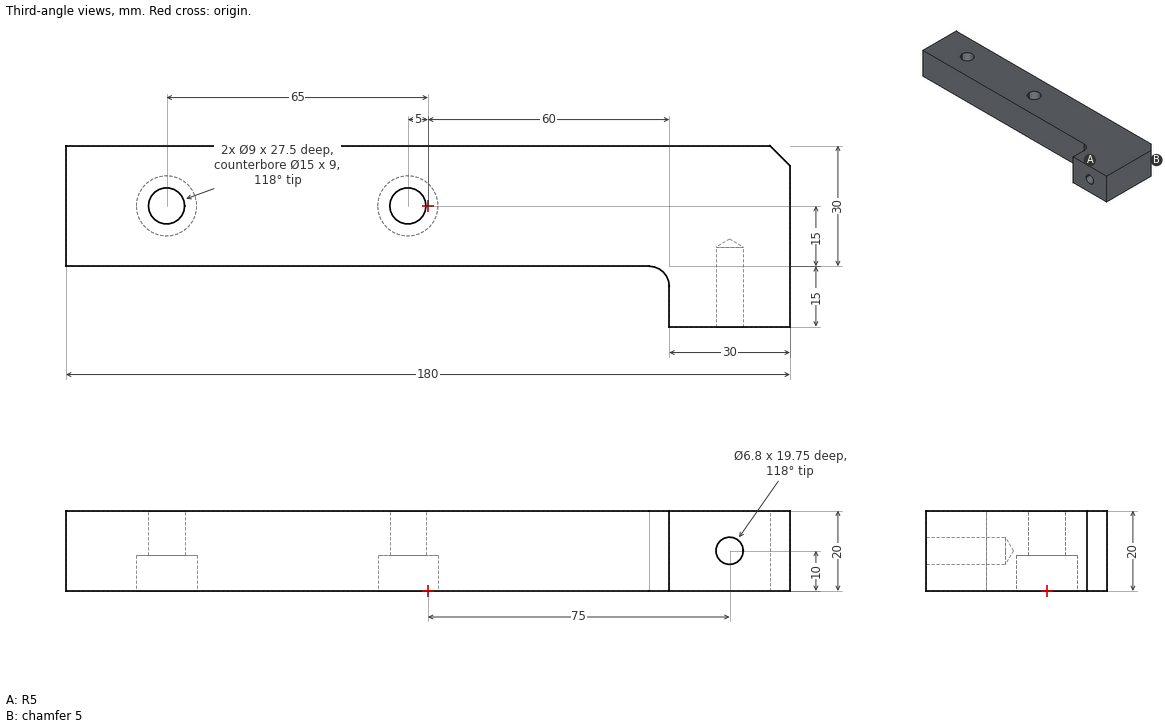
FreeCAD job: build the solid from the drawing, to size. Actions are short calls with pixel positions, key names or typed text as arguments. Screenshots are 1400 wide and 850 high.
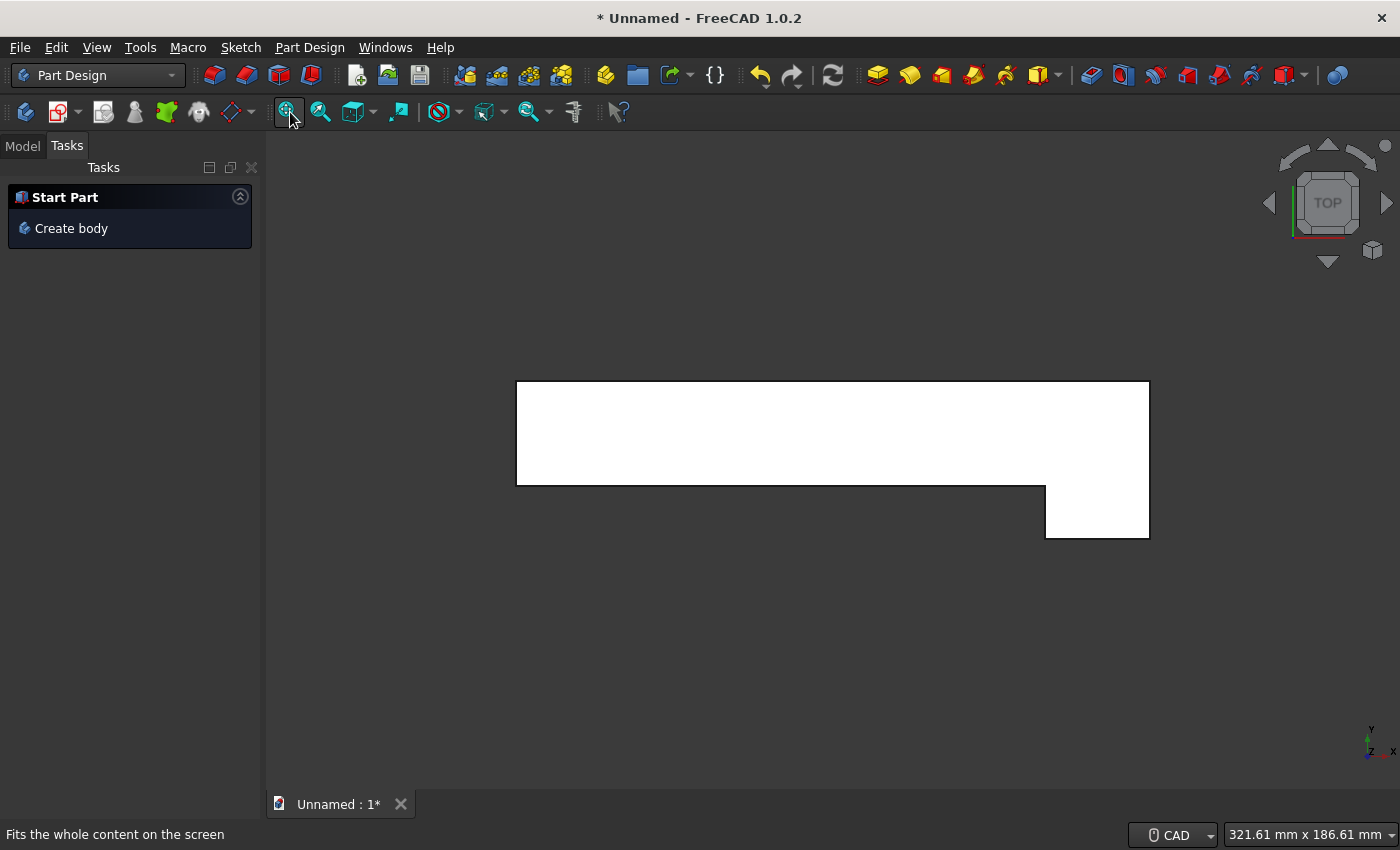
key(1)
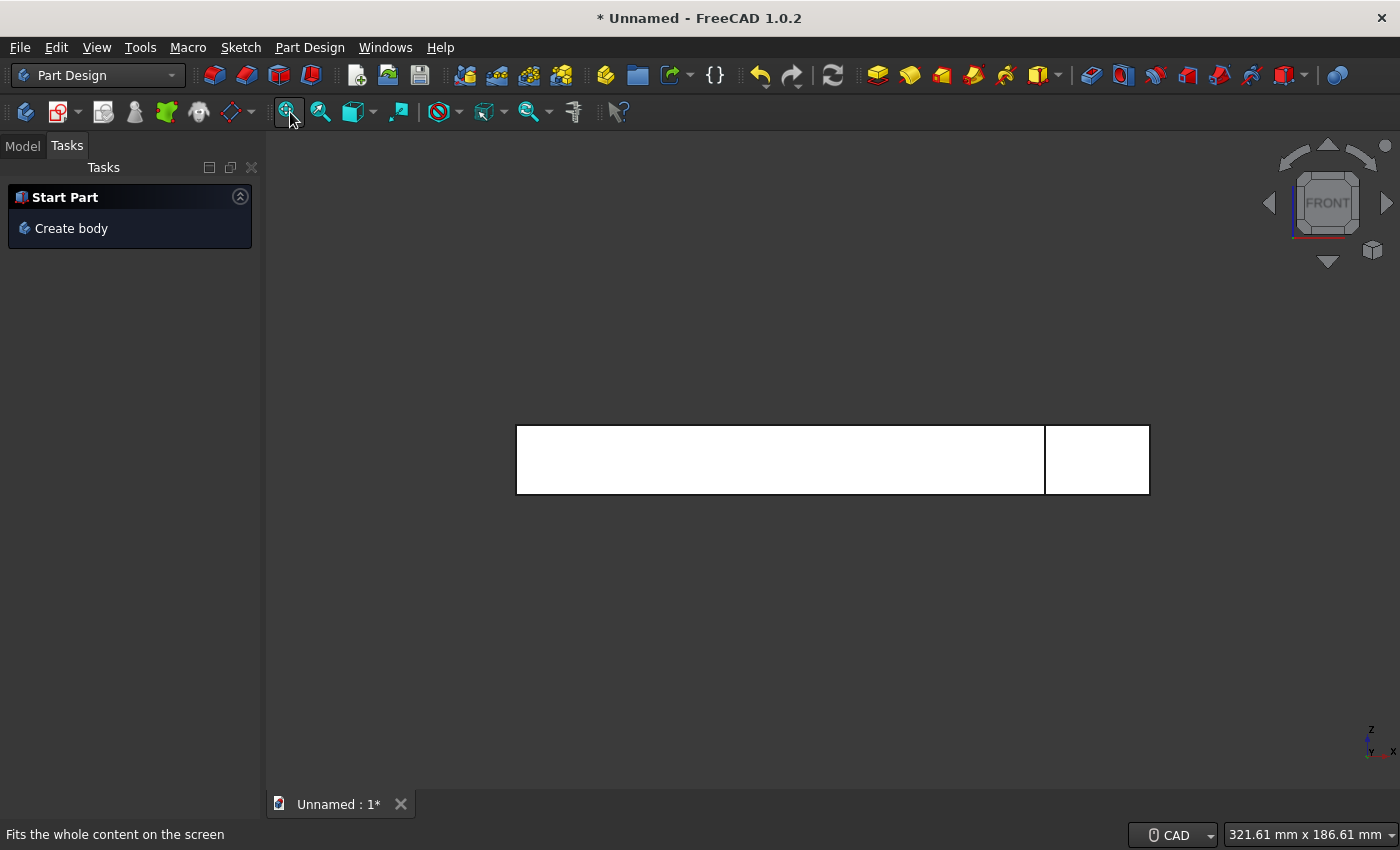
key(3)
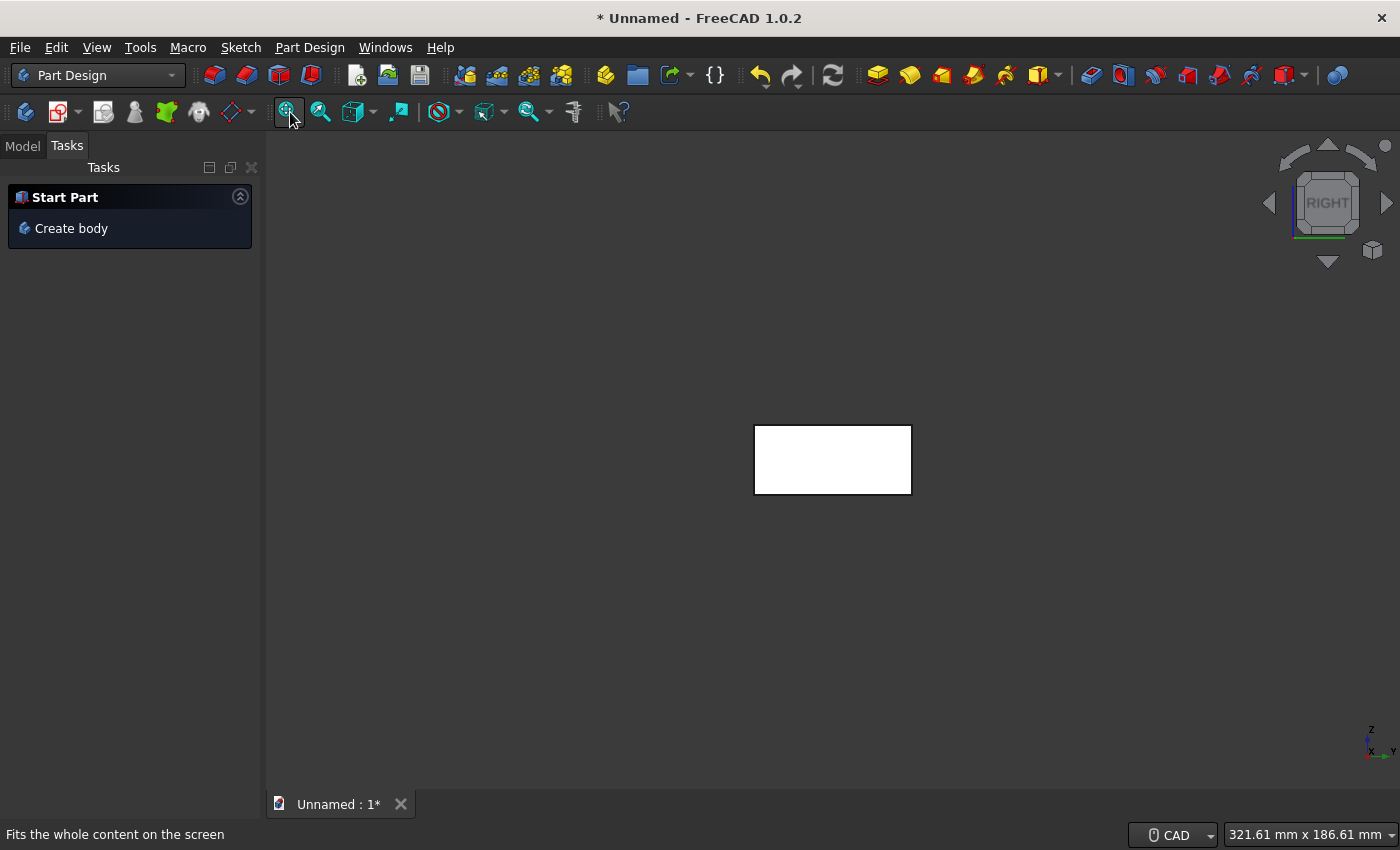
click(290, 112)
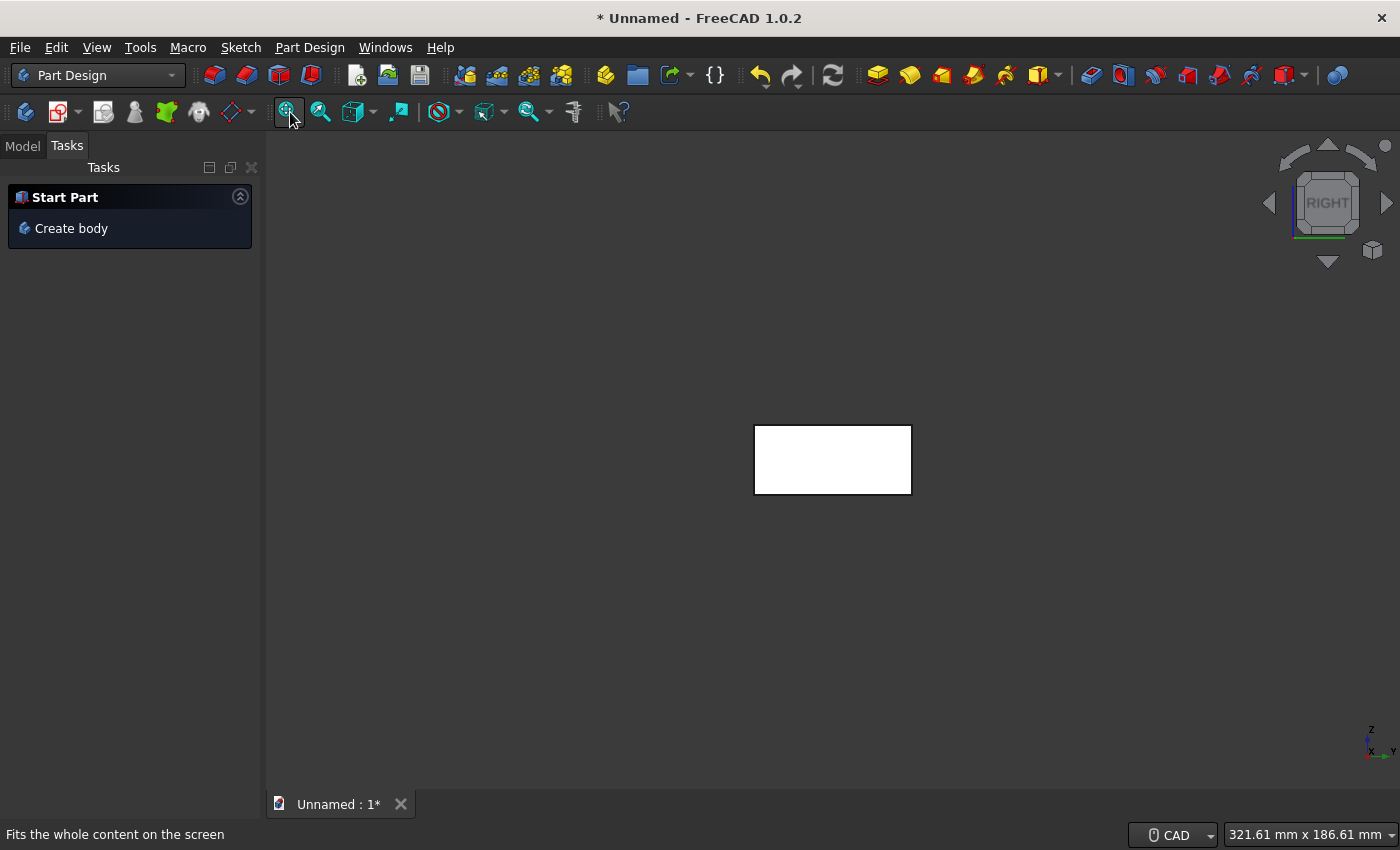
key(5)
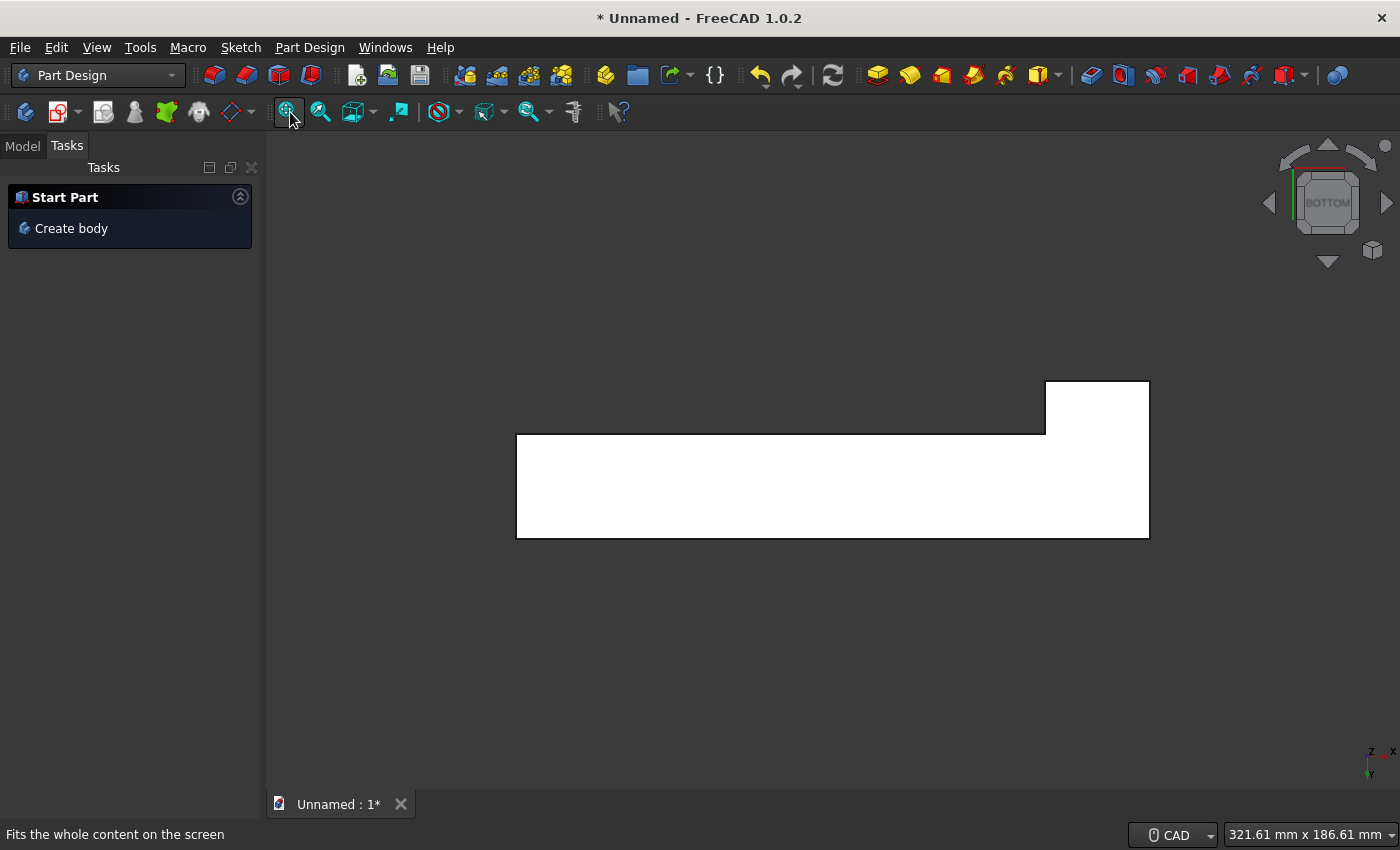
key(4)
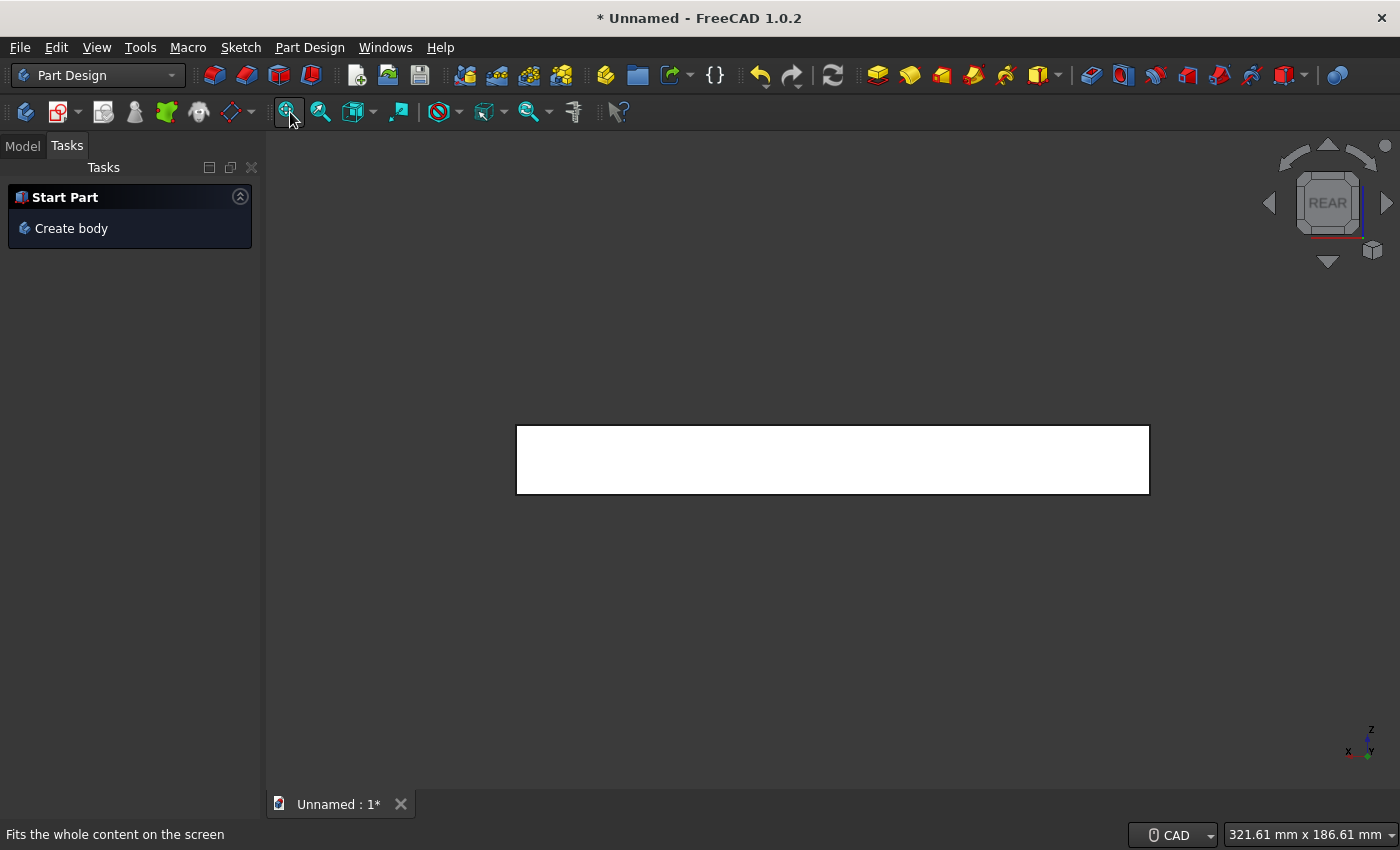
key(6)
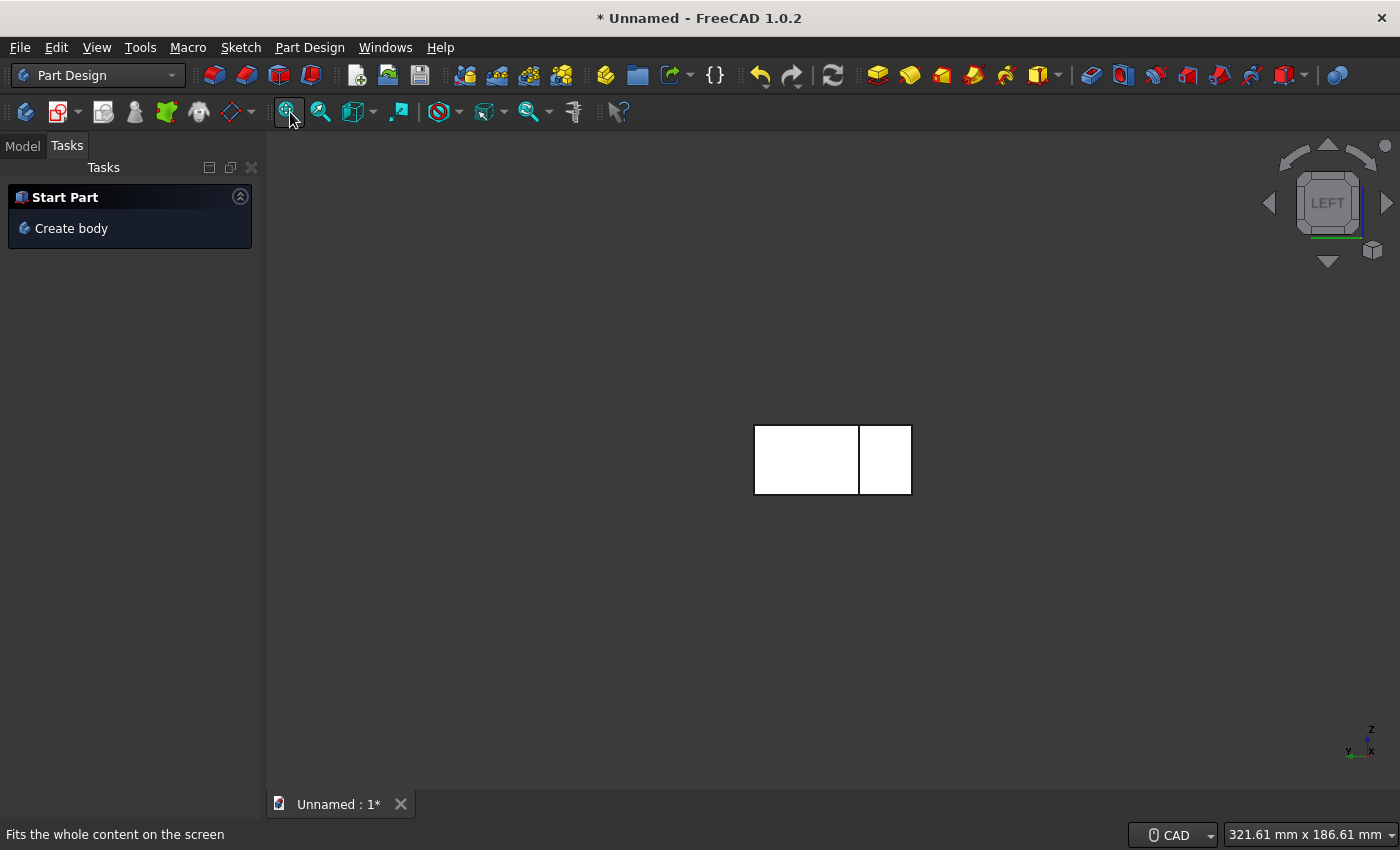
click(290, 112)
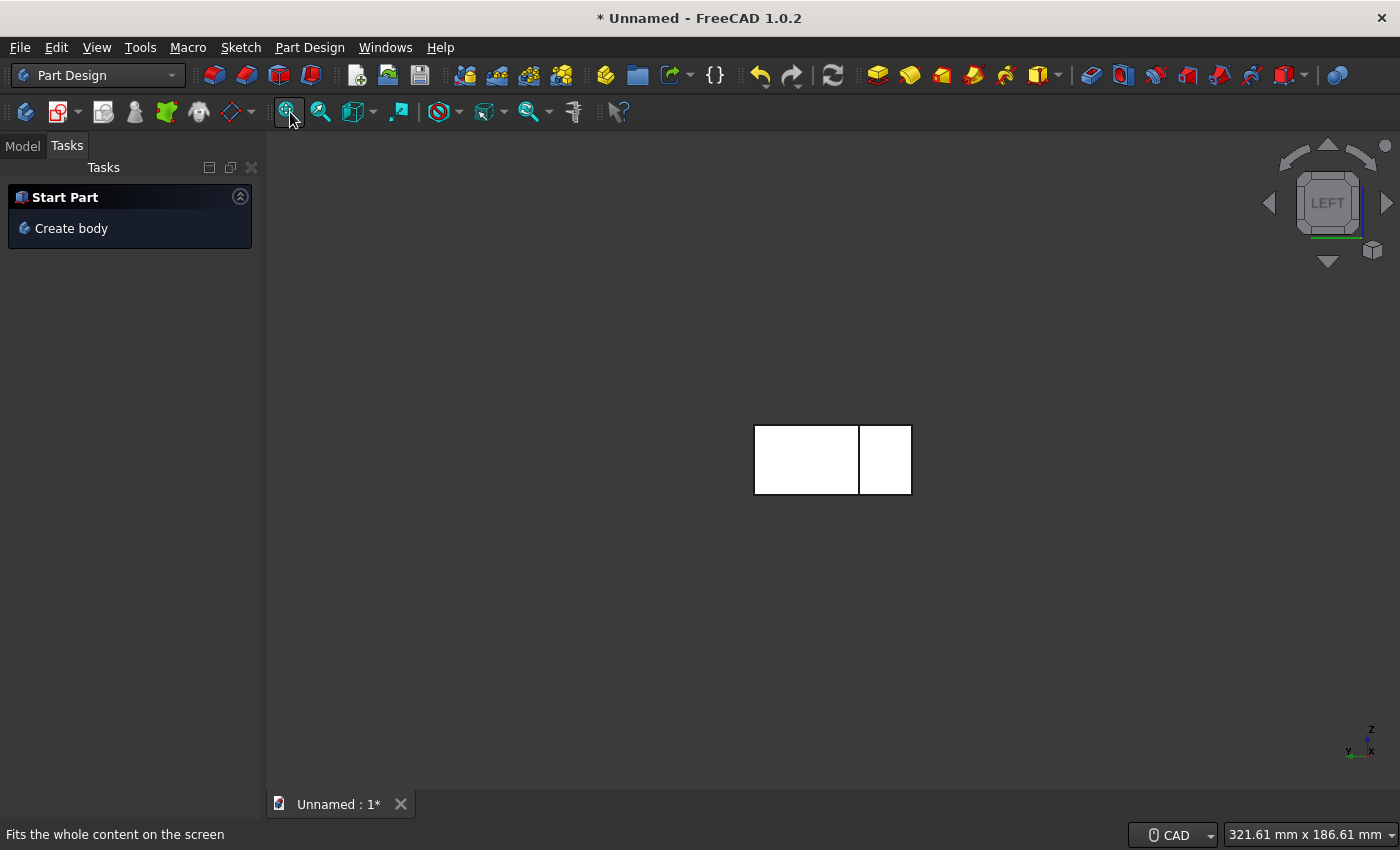
key(v)
key(3)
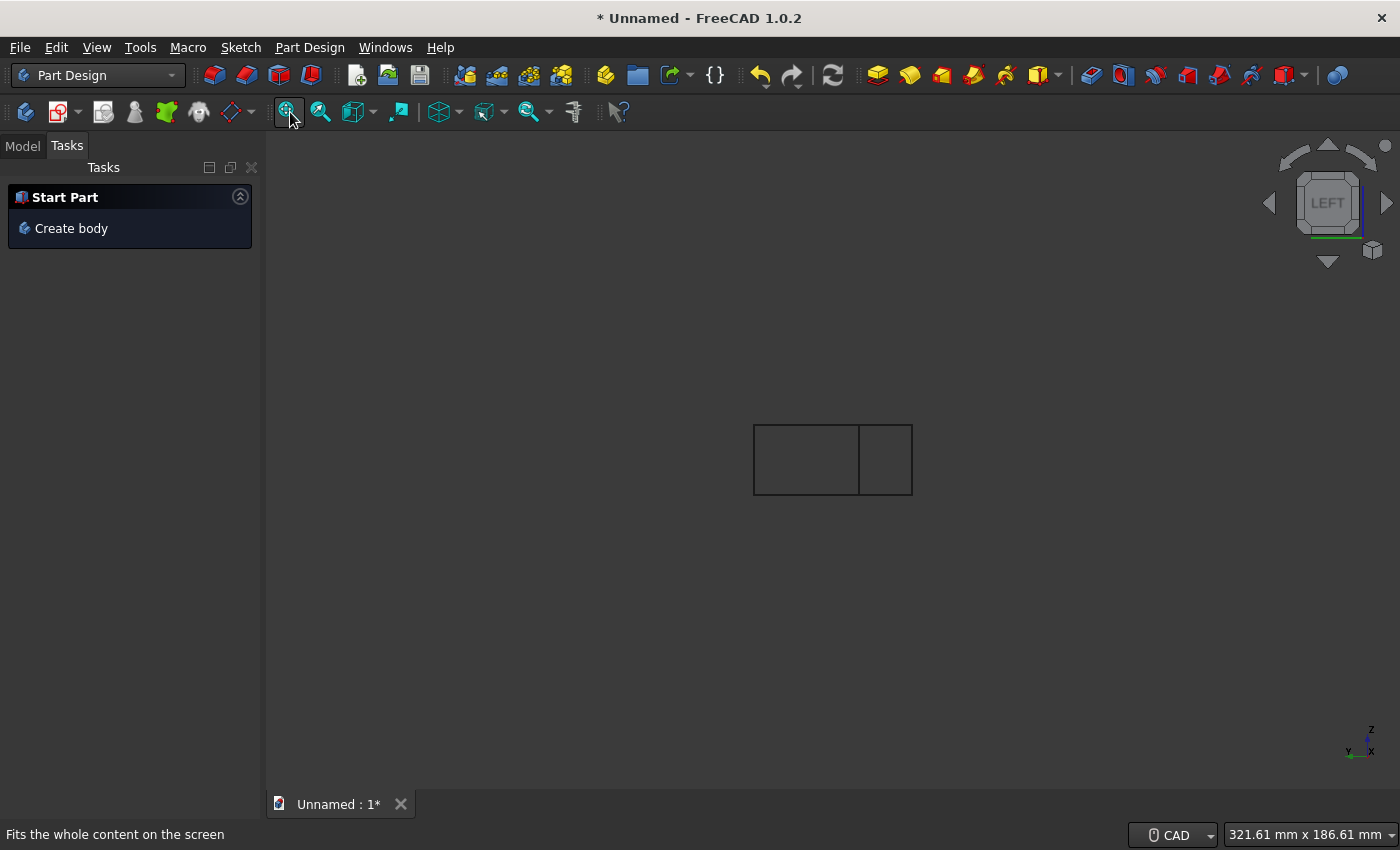
key(0)